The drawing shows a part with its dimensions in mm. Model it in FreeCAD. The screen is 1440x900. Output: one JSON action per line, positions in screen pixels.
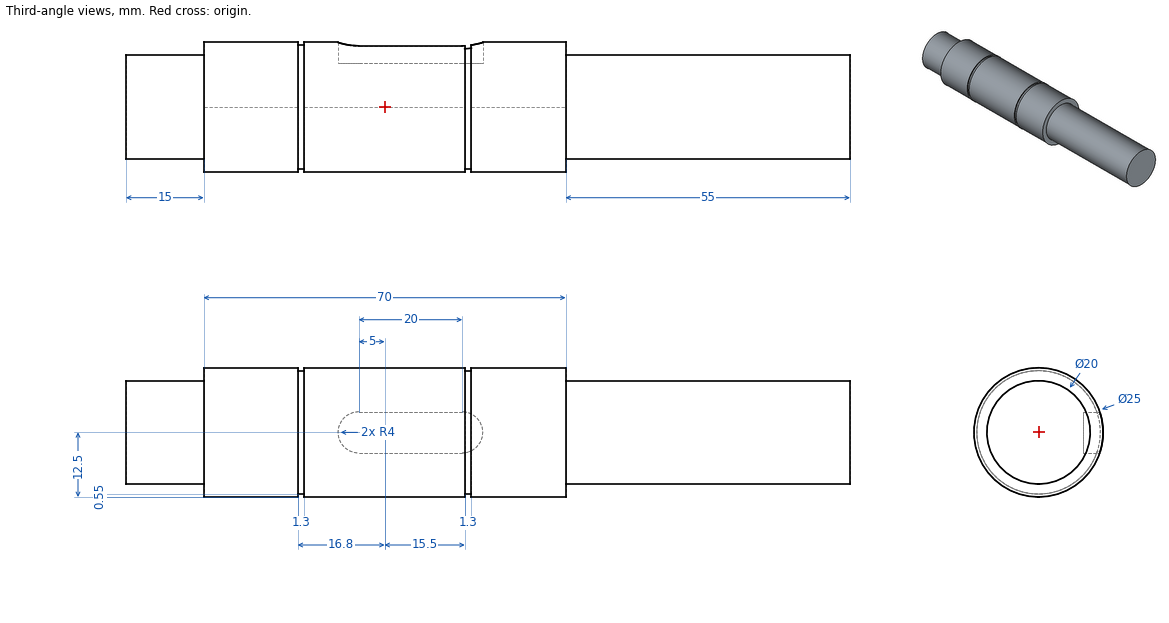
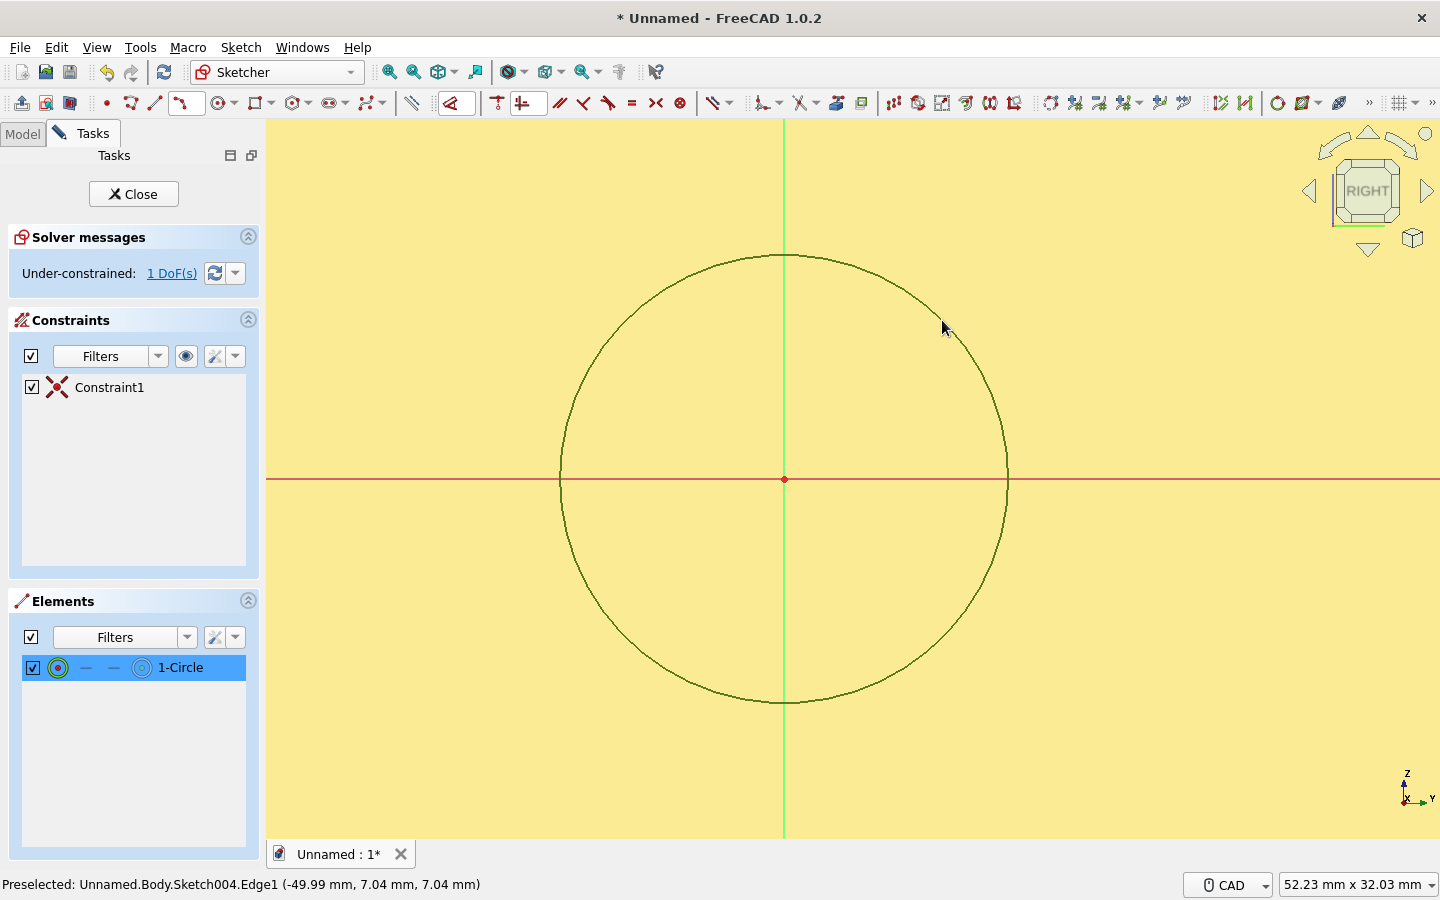
{"action": "key", "text": "k o"}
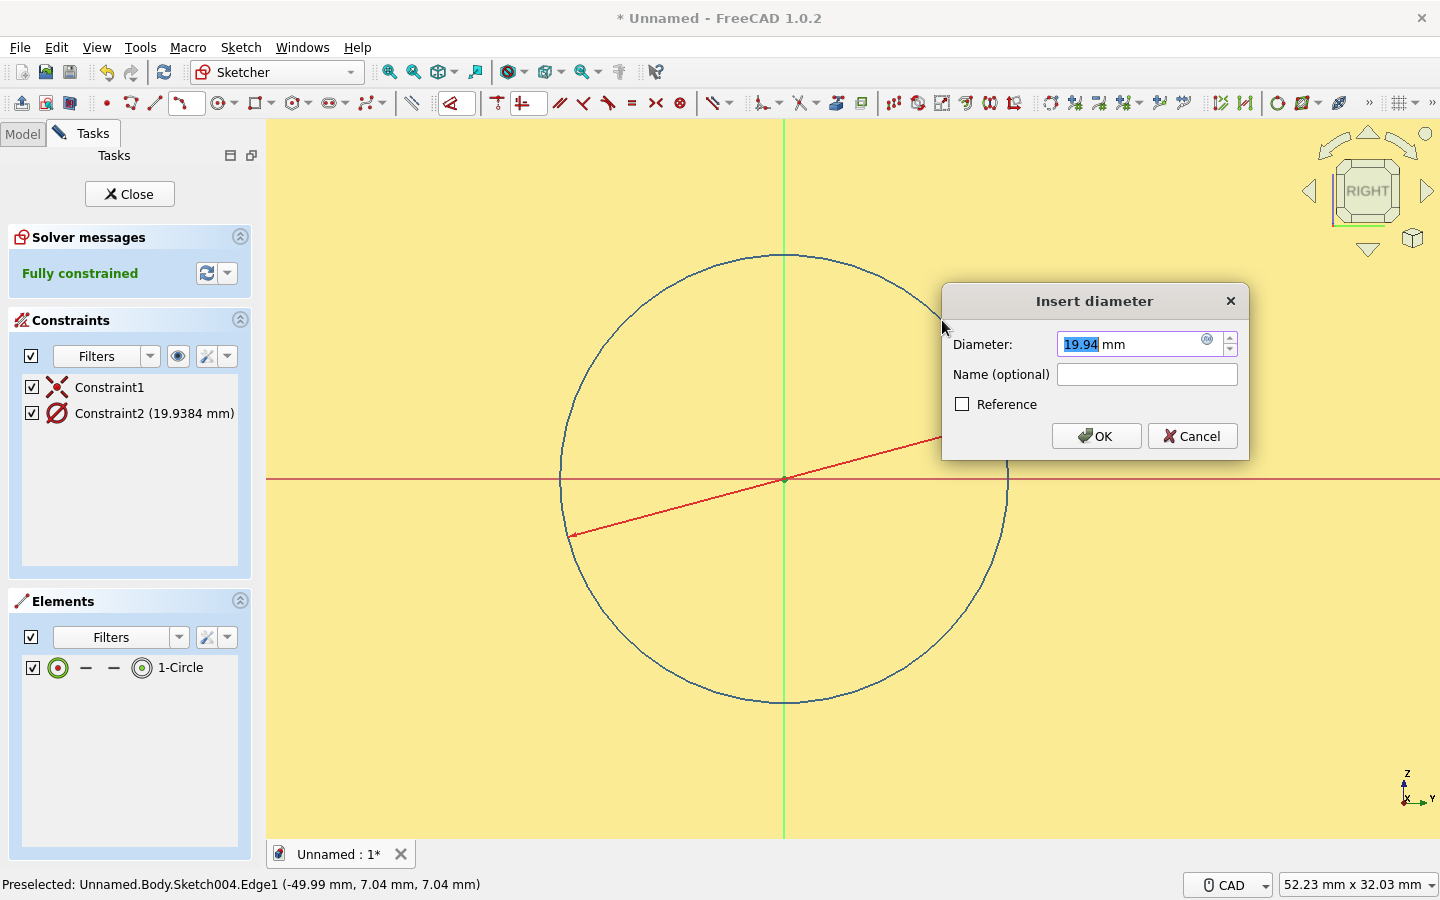
{"action": "type", "text": "20"}
{"action": "key", "text": "Return"}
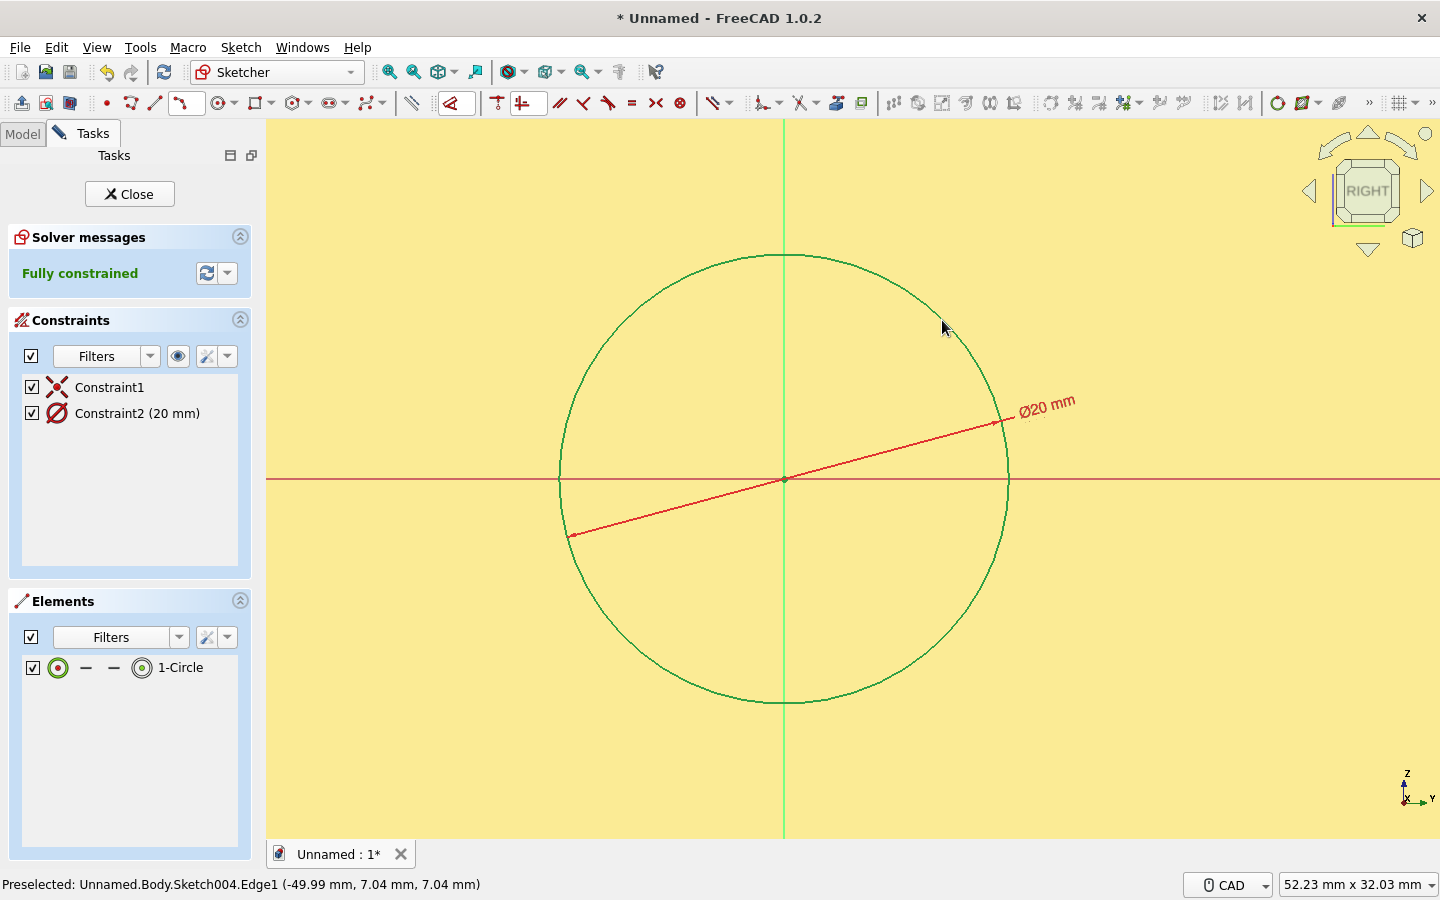
{"action": "left_click", "coordinate": [130, 194]}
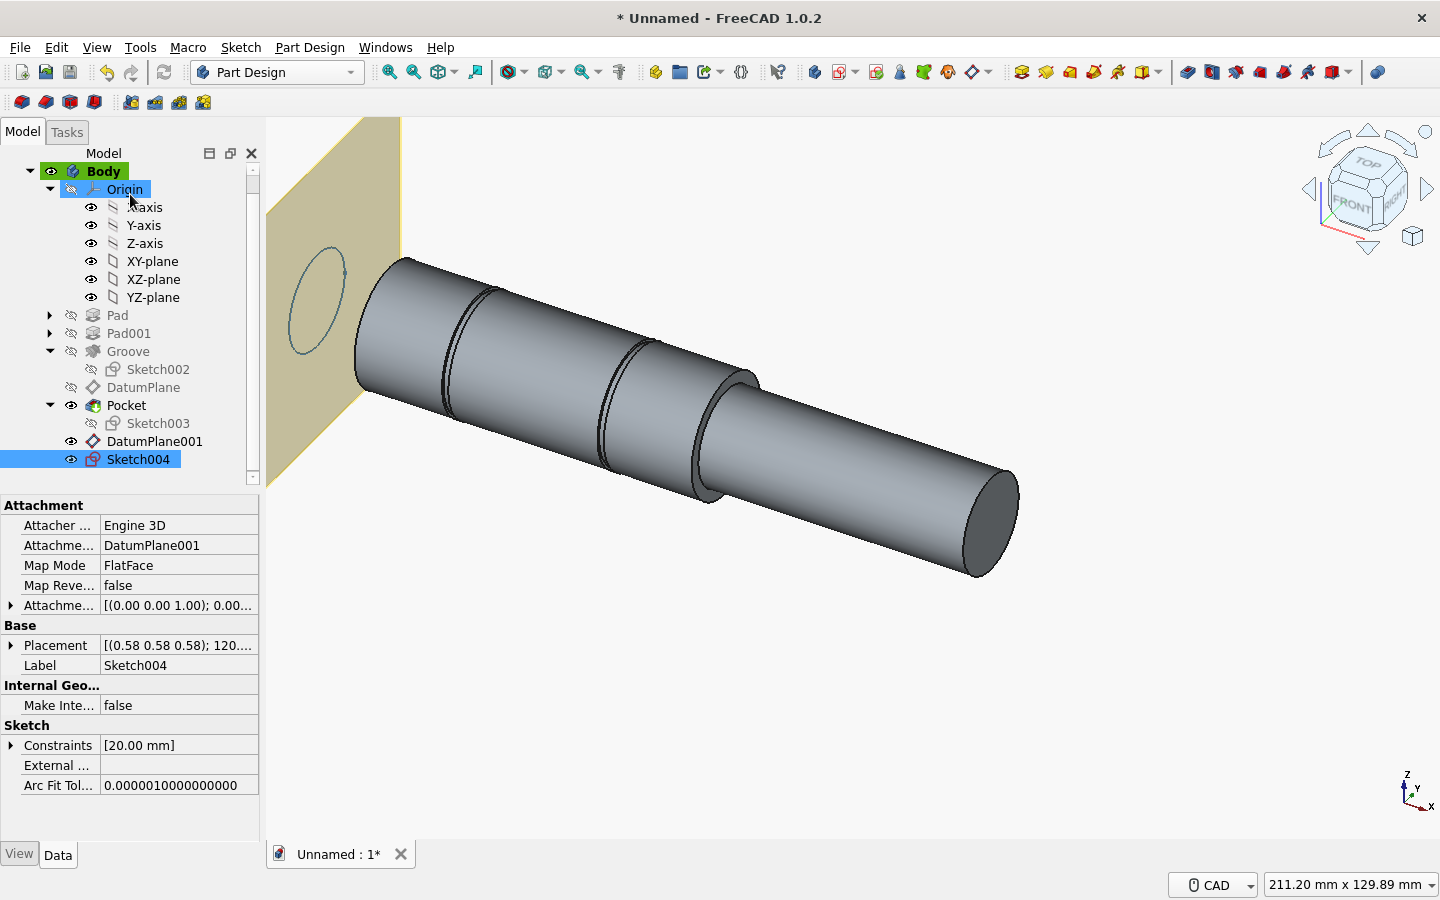
{"action": "left_click", "coordinate": [1022, 72]}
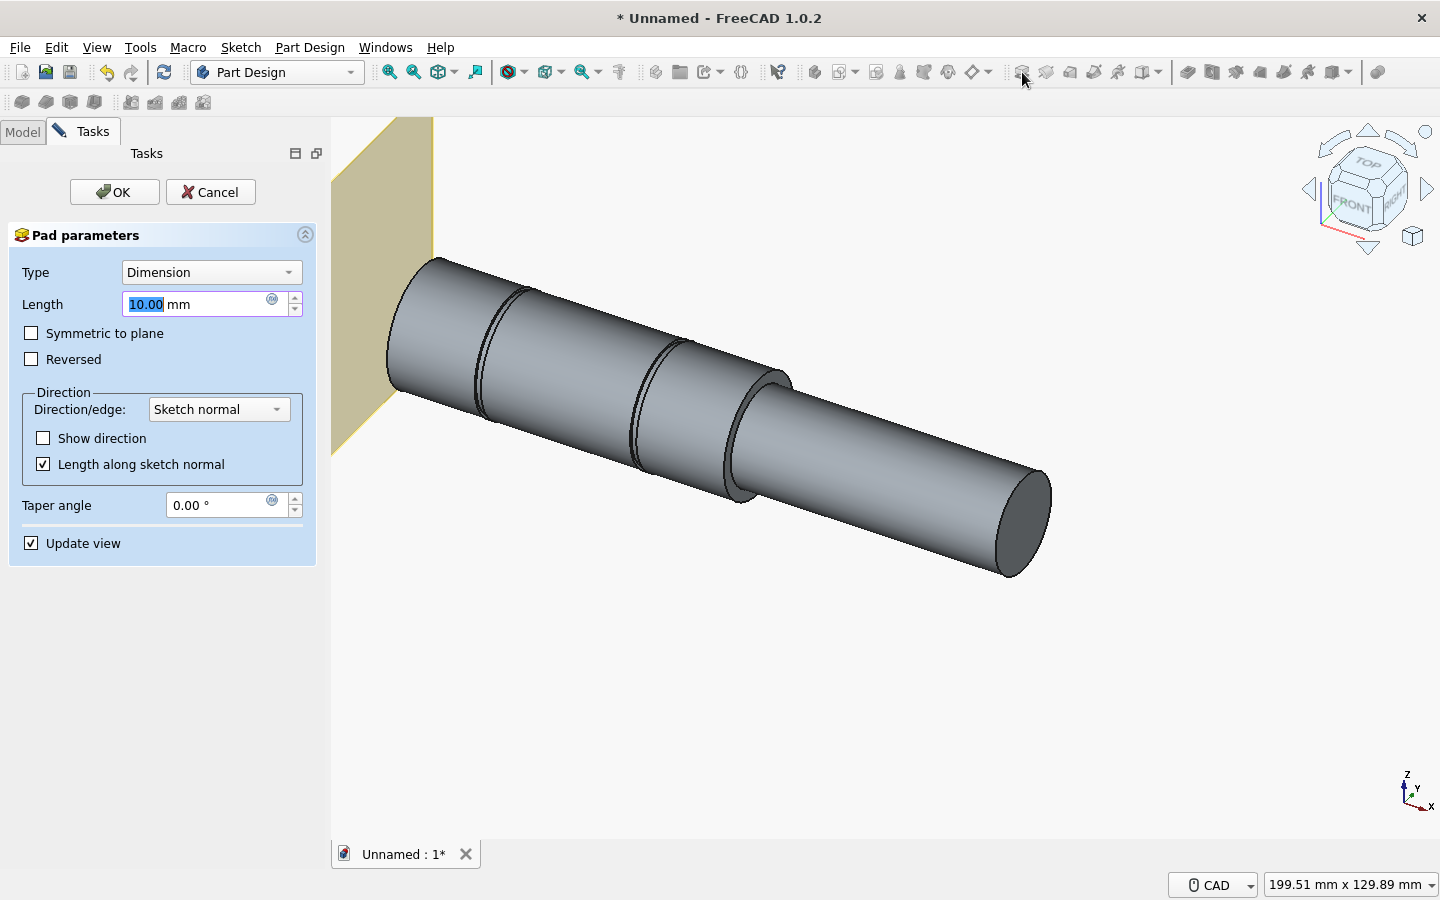
{"action": "type", "text": "15"}
{"action": "key", "text": "Tab"}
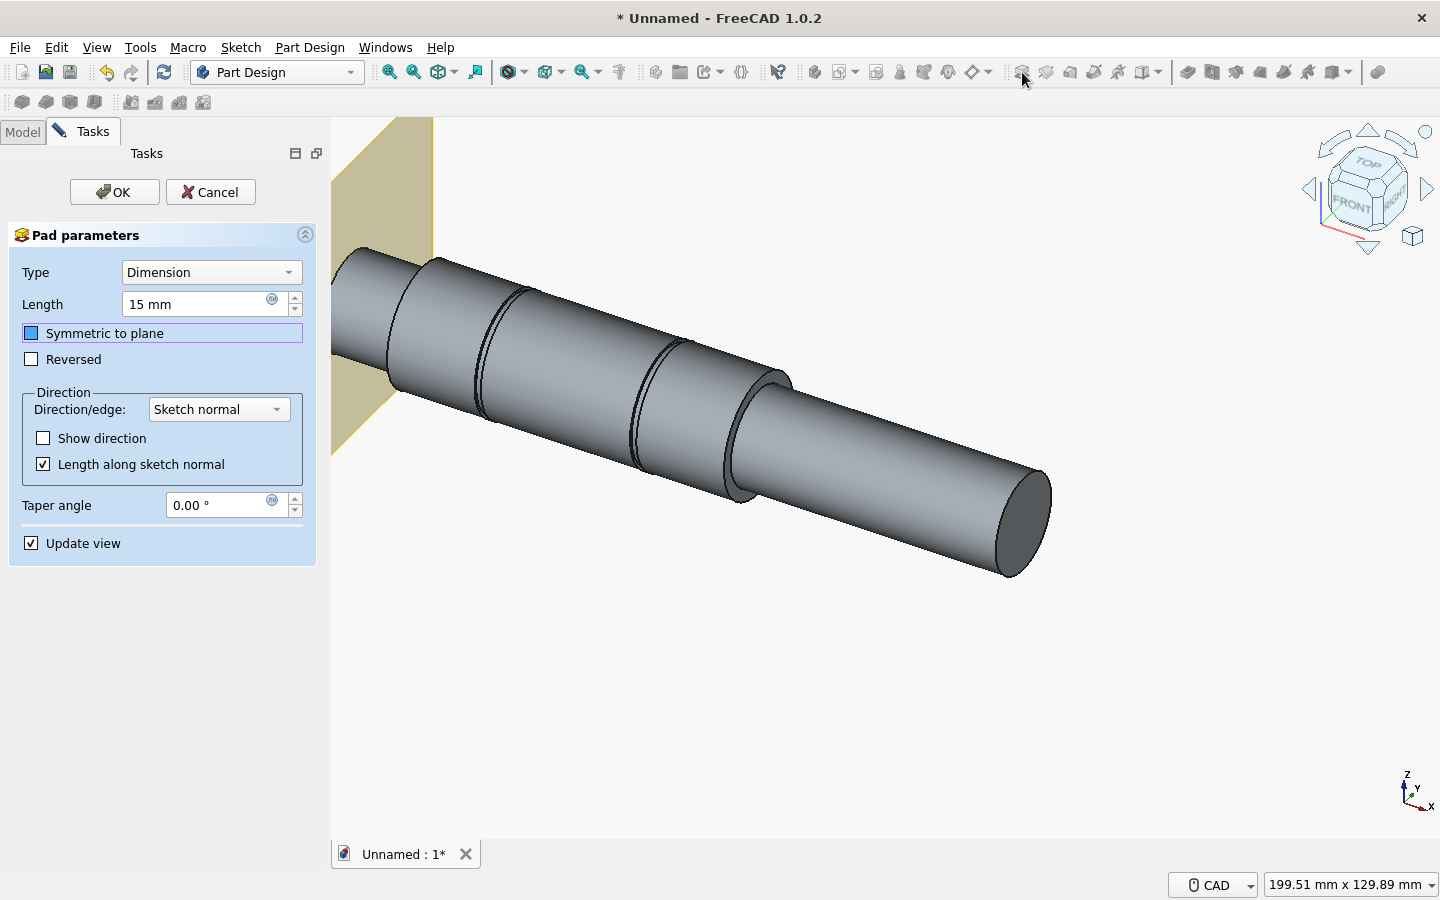
{"action": "left_click", "coordinate": [115, 192]}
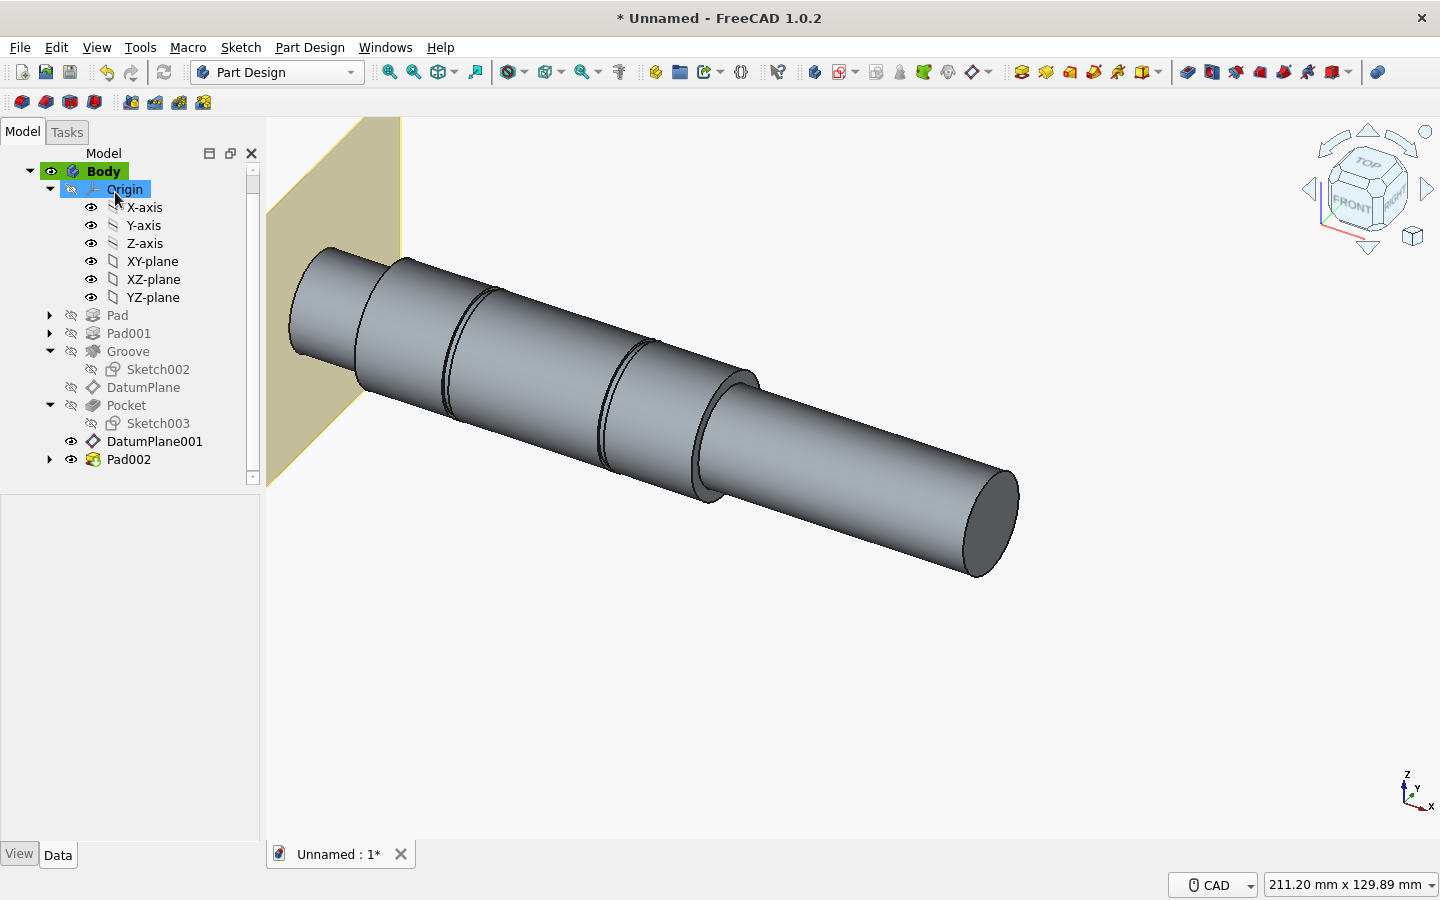
{"action": "left_click", "coordinate": [116, 441]}
{"action": "key", "text": "space"}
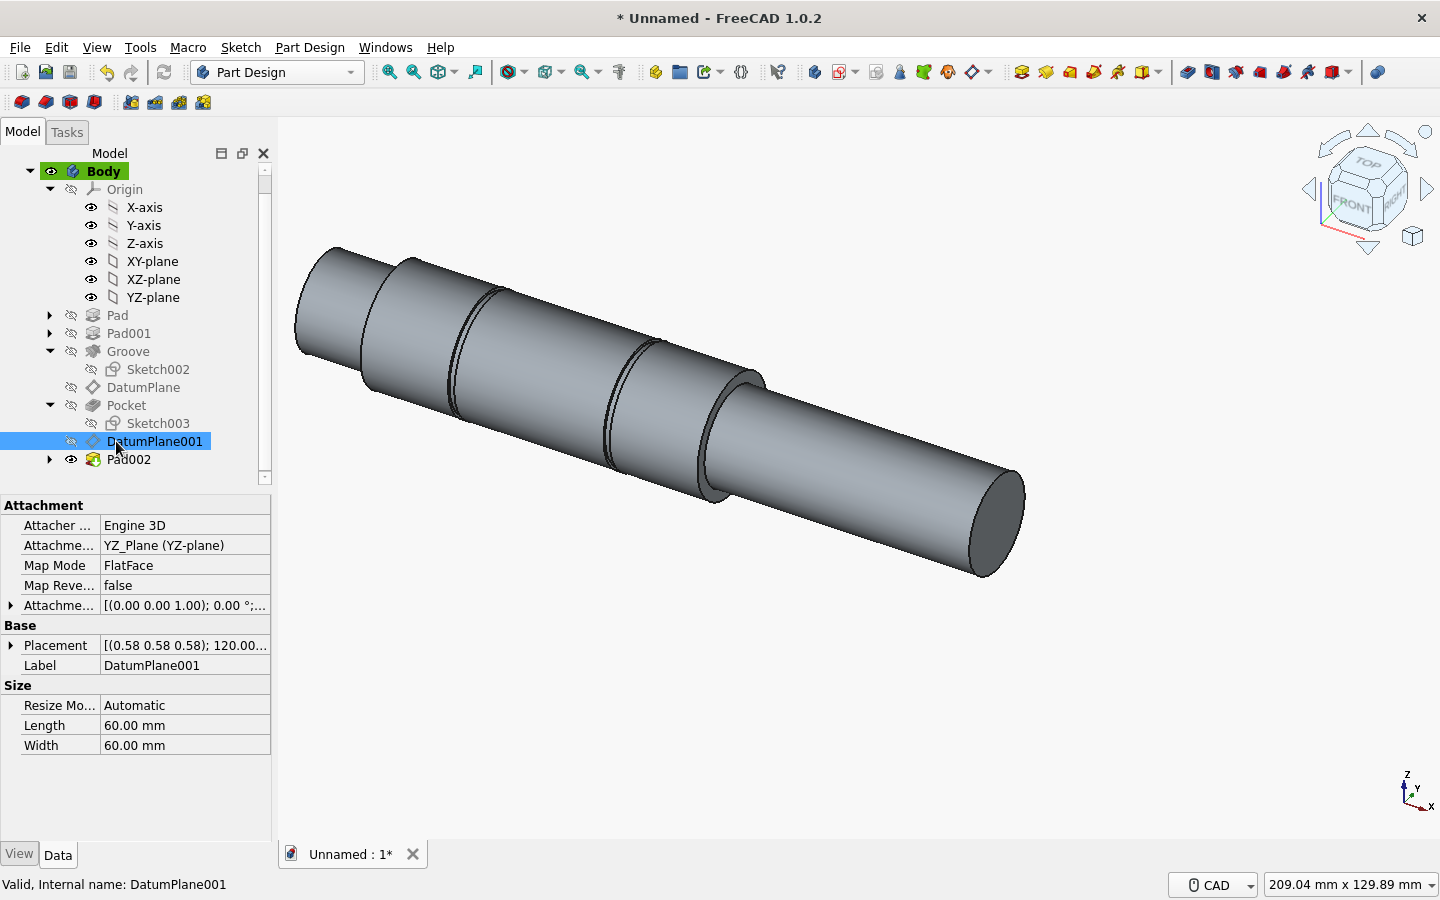
{"action": "key", "text": "0"}